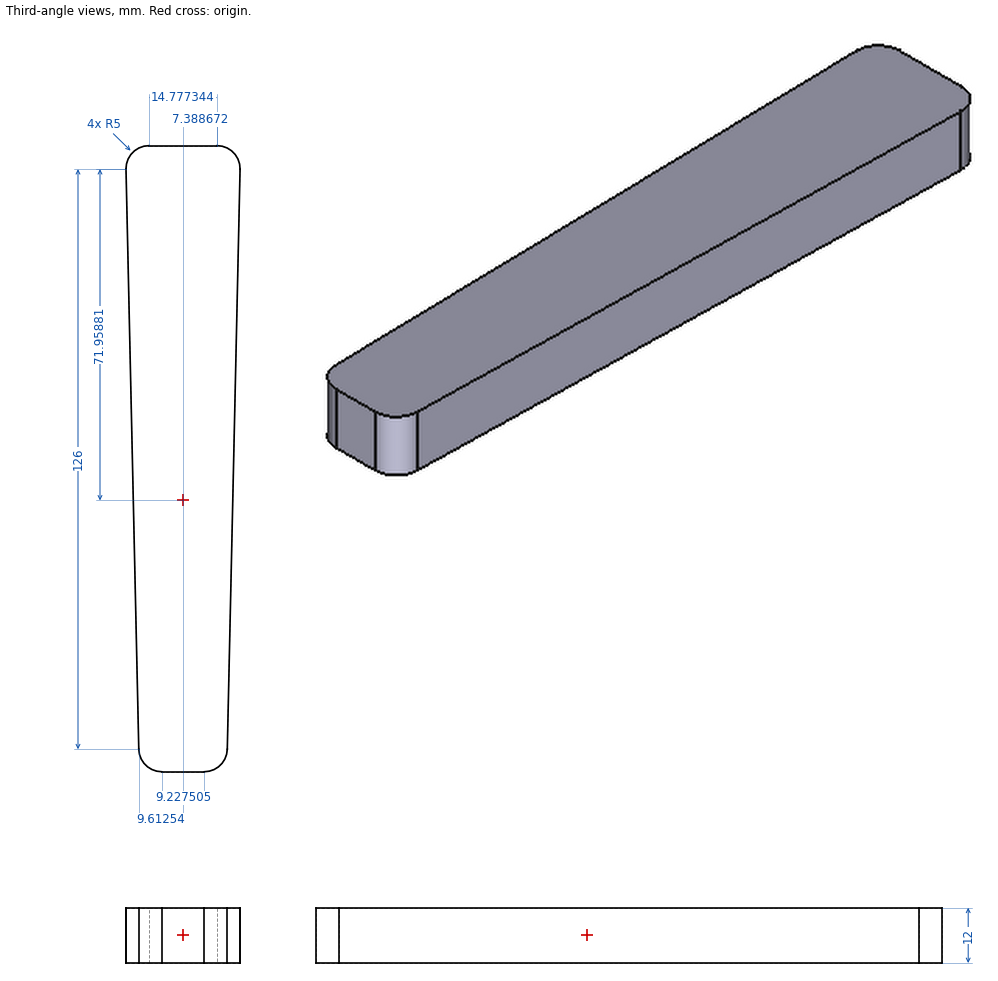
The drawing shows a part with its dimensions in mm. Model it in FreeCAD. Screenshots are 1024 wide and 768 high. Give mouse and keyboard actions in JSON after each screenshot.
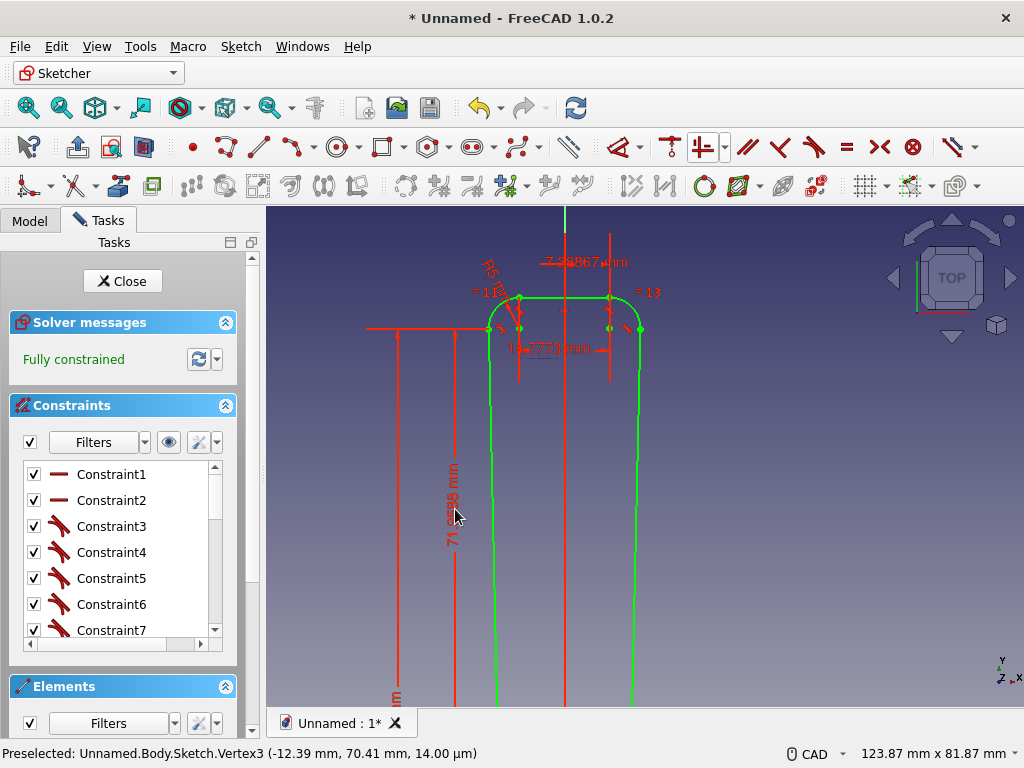
{"action": "left_click", "coordinate": [123, 281]}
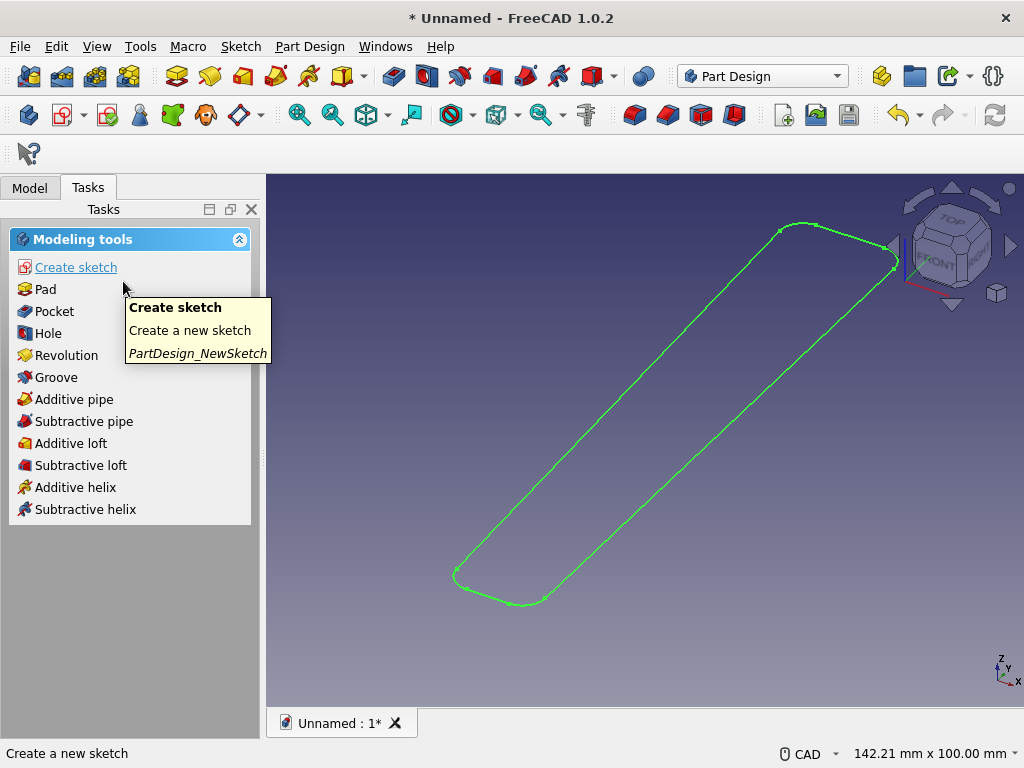
{"action": "left_click", "coordinate": [177, 76]}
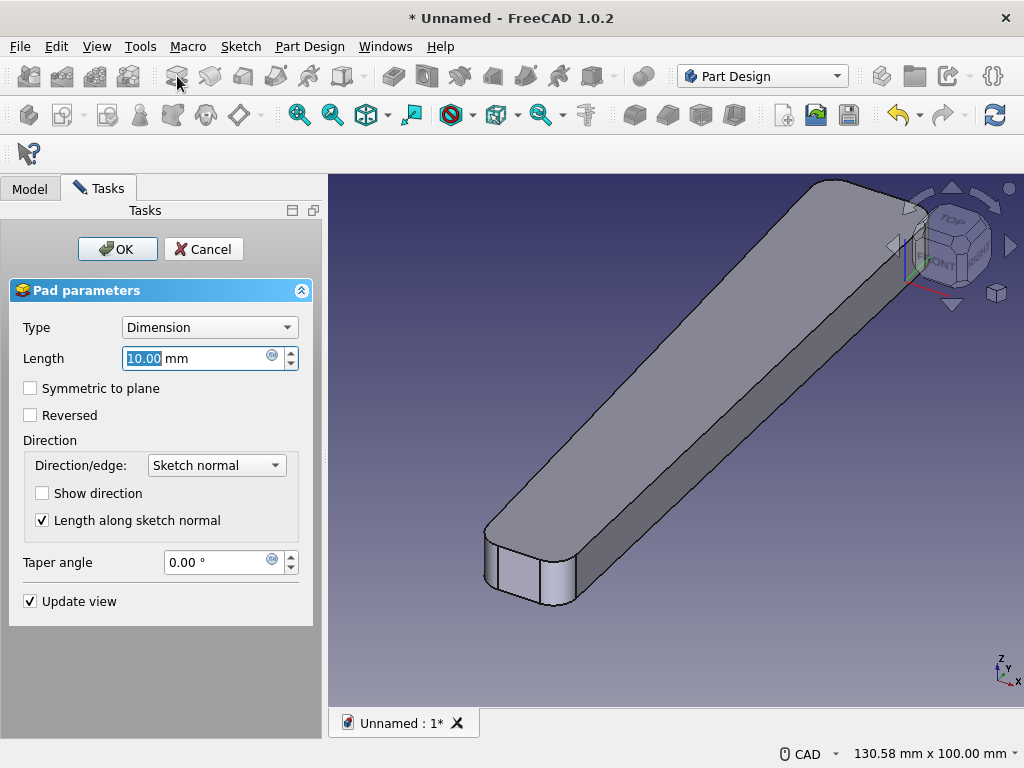
{"action": "type", "text": "12"}
{"action": "key", "text": "Tab"}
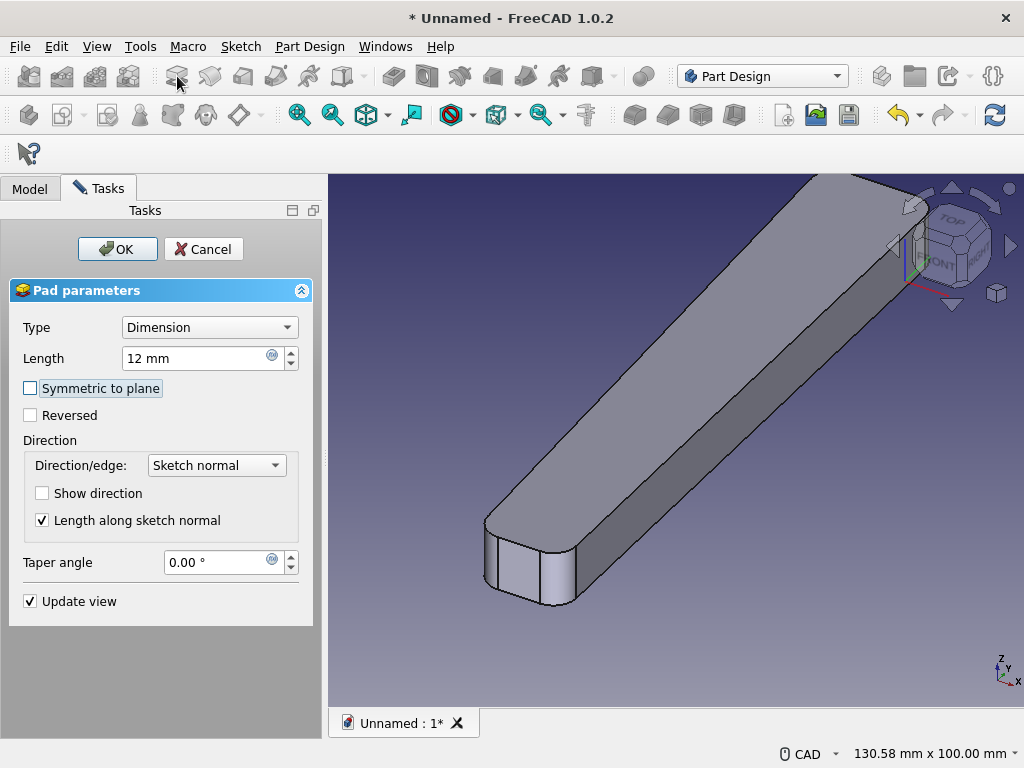
{"action": "left_click", "coordinate": [31, 388]}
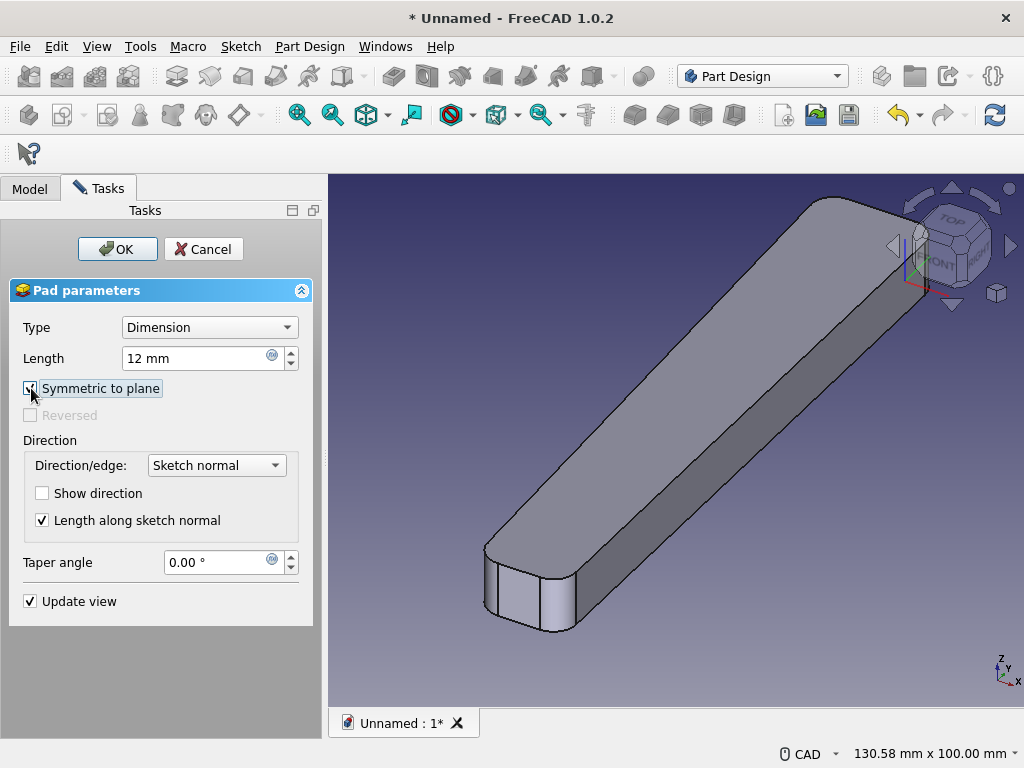
{"action": "left_click", "coordinate": [118, 249]}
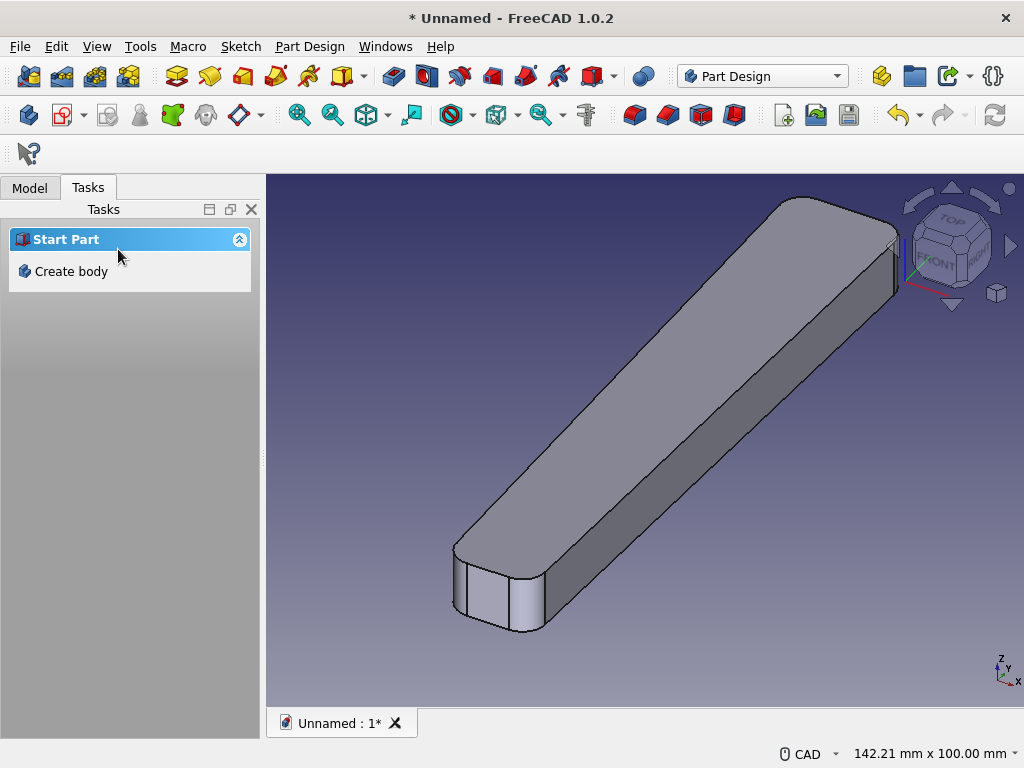
{"action": "key", "text": "0"}